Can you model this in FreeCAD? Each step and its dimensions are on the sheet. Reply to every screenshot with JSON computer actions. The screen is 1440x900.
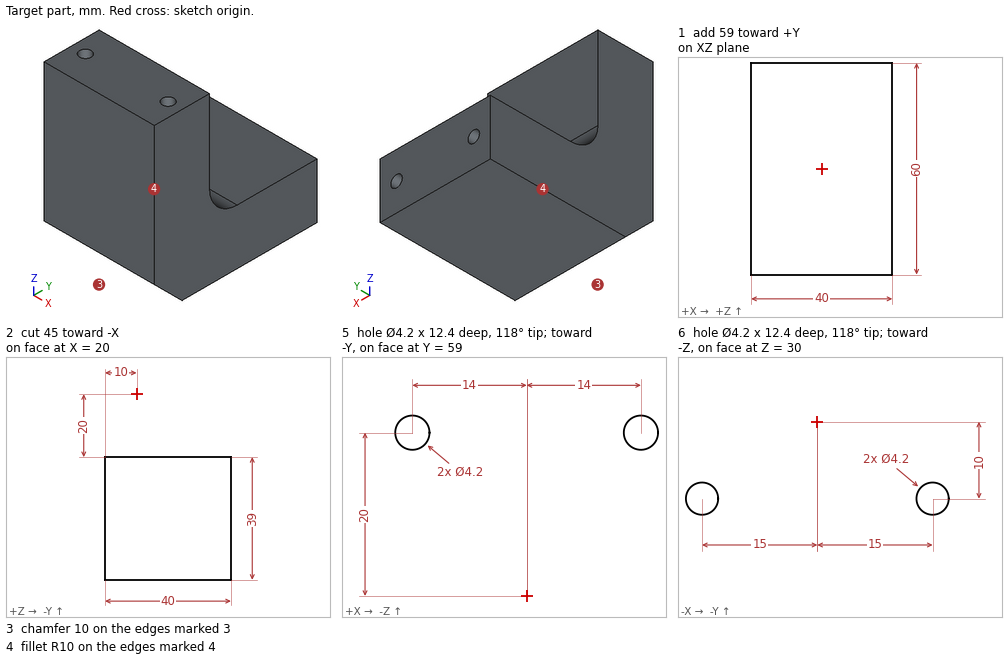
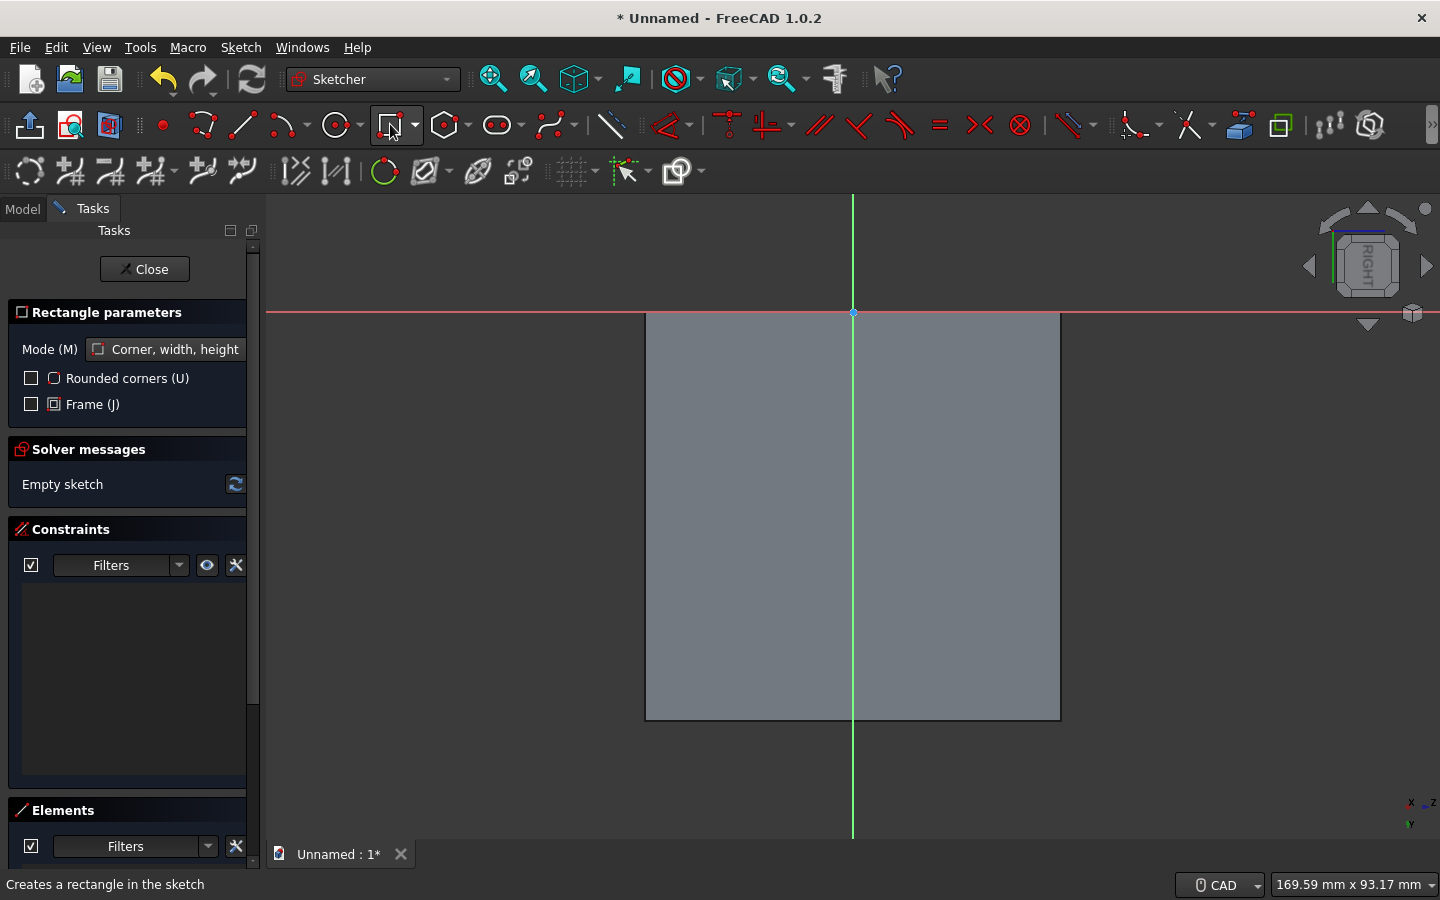
{"action": "left_click", "coordinate": [784, 451]}
{"action": "mouse_move", "coordinate": [1061, 721]}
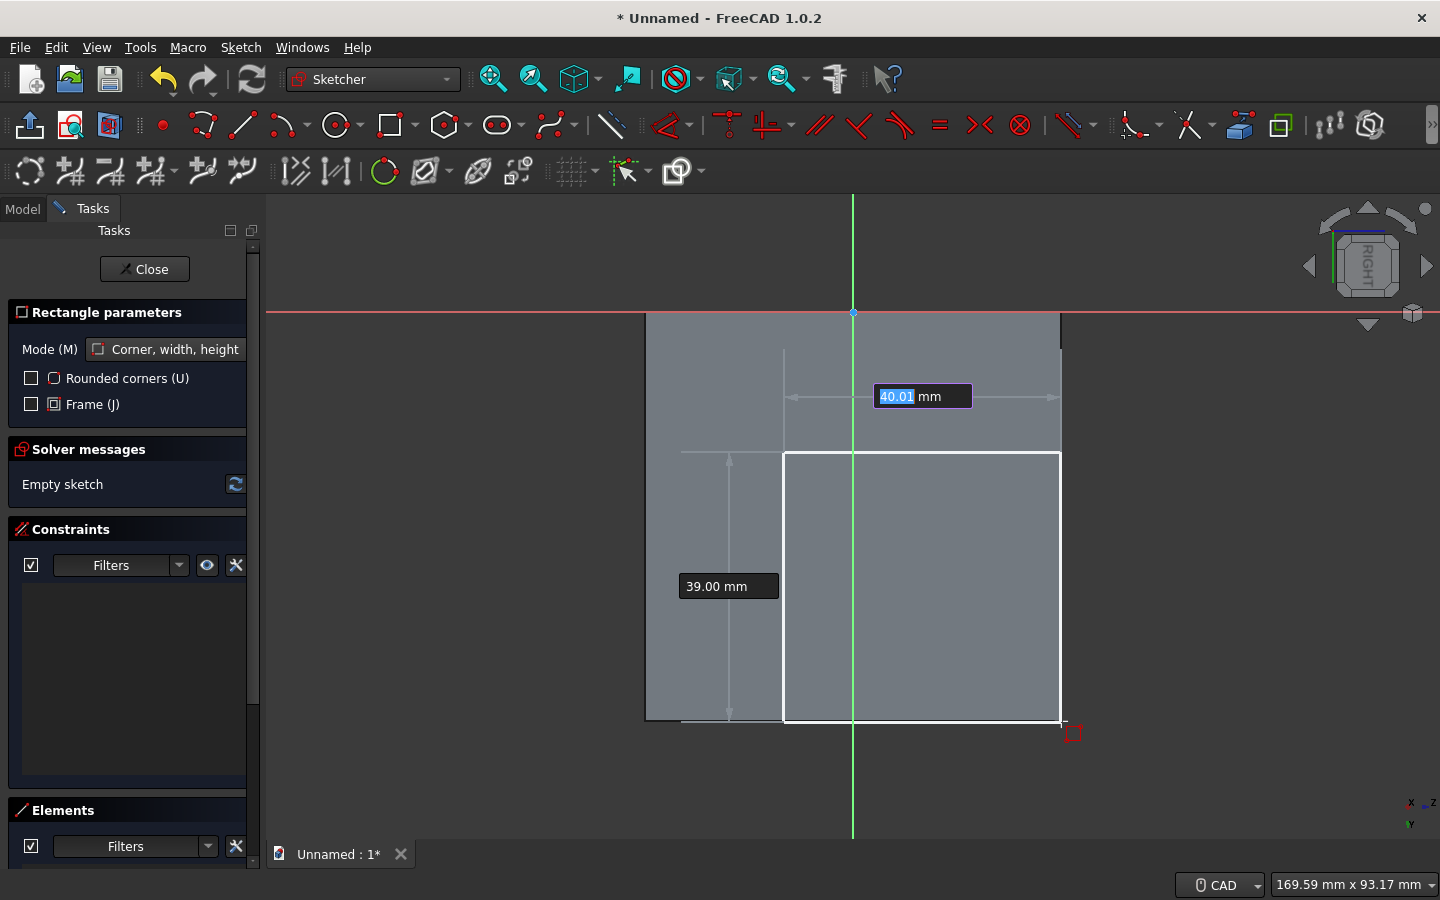
{"action": "type", "text": "40"}
{"action": "key", "text": "Tab"}
{"action": "type", "text": "39"}
{"action": "key", "text": "Return"}
{"action": "key", "text": "Escape"}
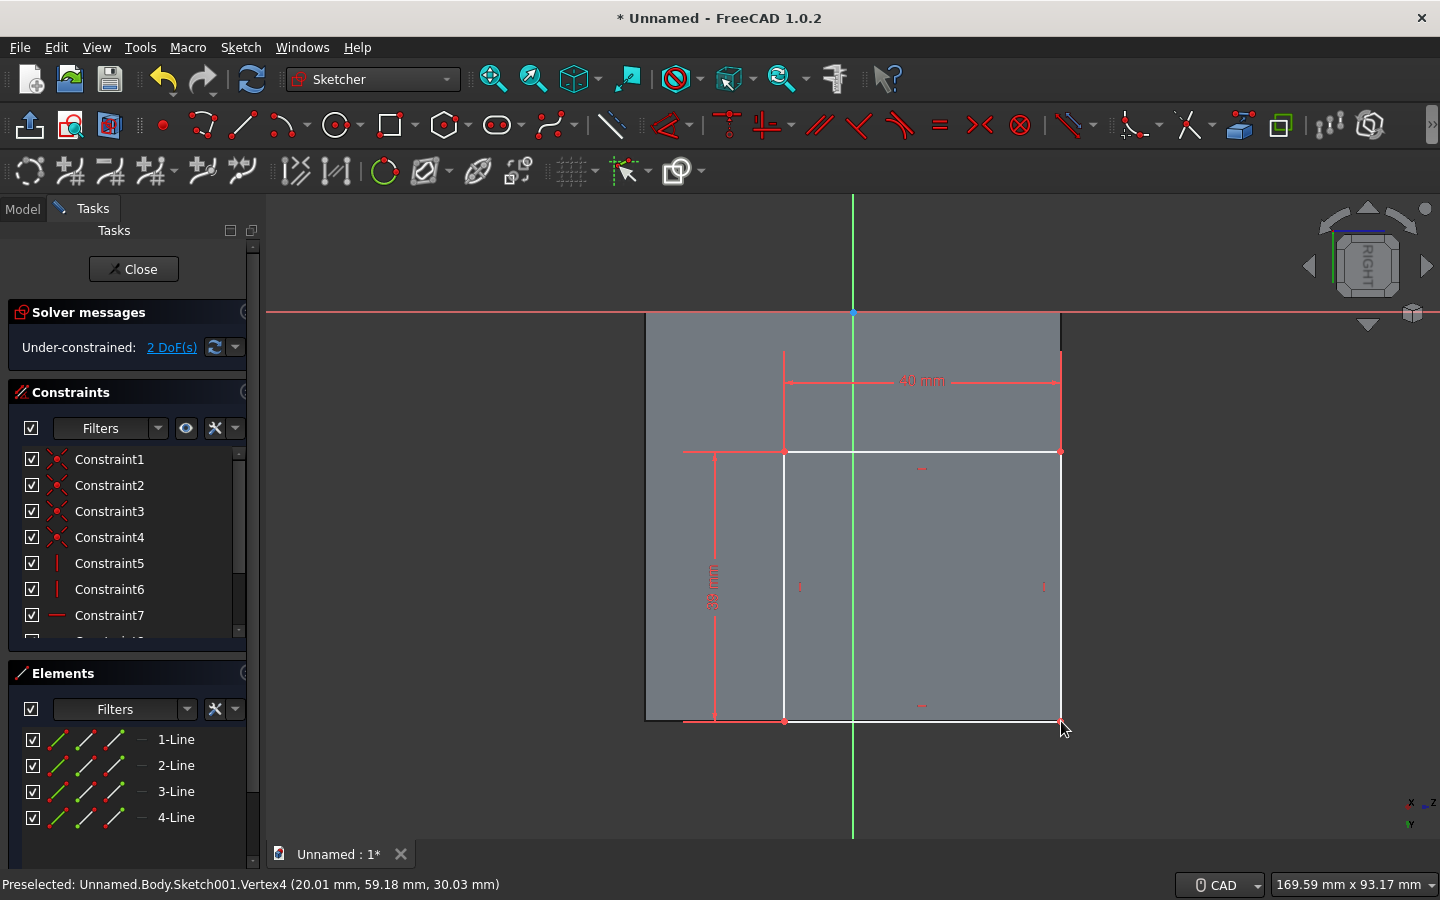
{"action": "left_click", "coordinate": [666, 126]}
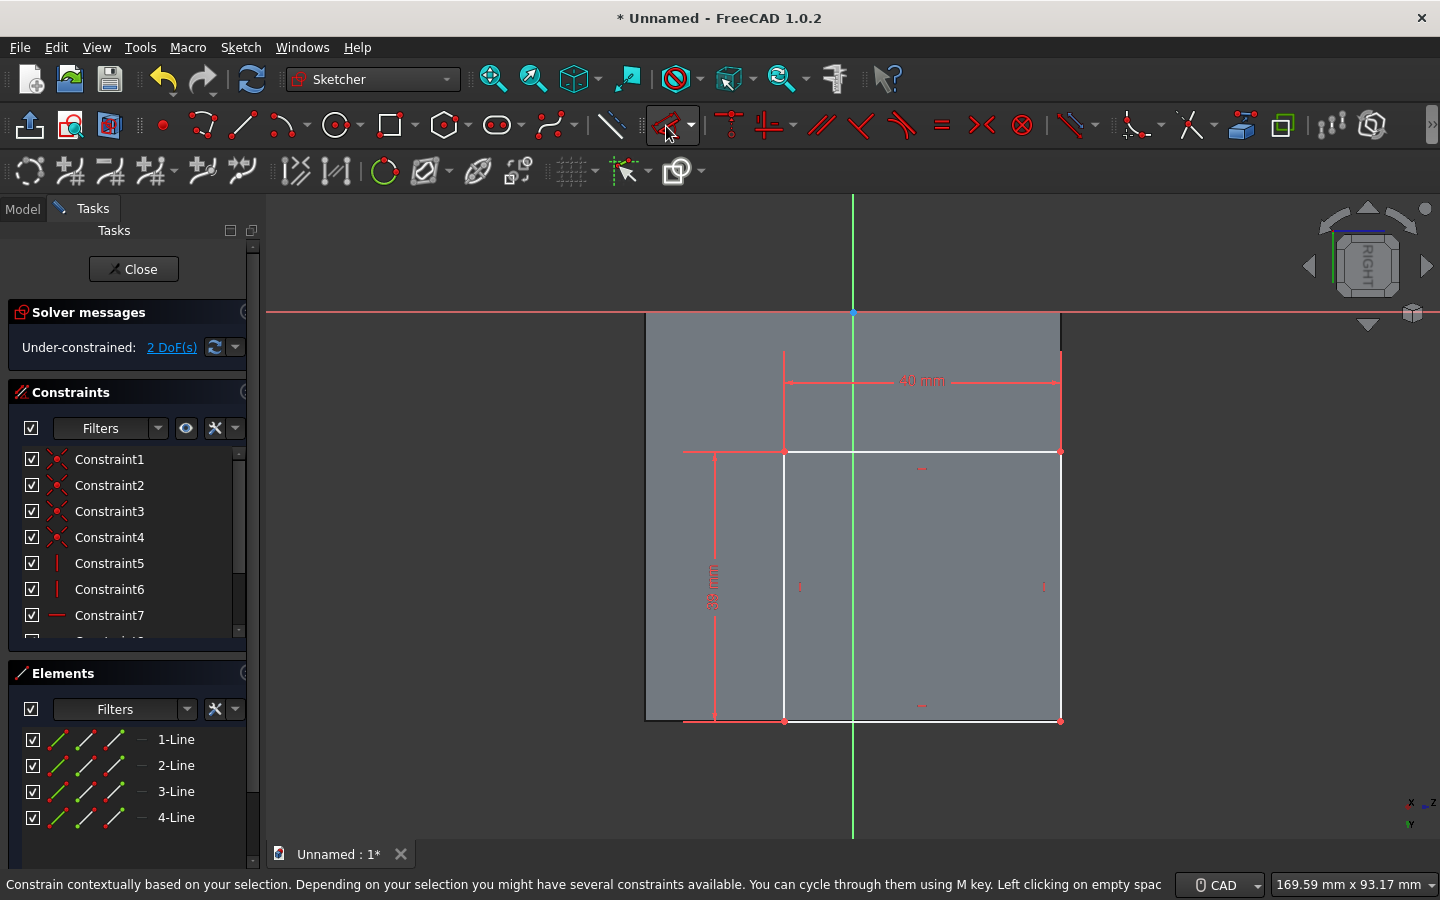
{"action": "left_click", "coordinate": [784, 452]}
{"action": "left_click", "coordinate": [818, 278]}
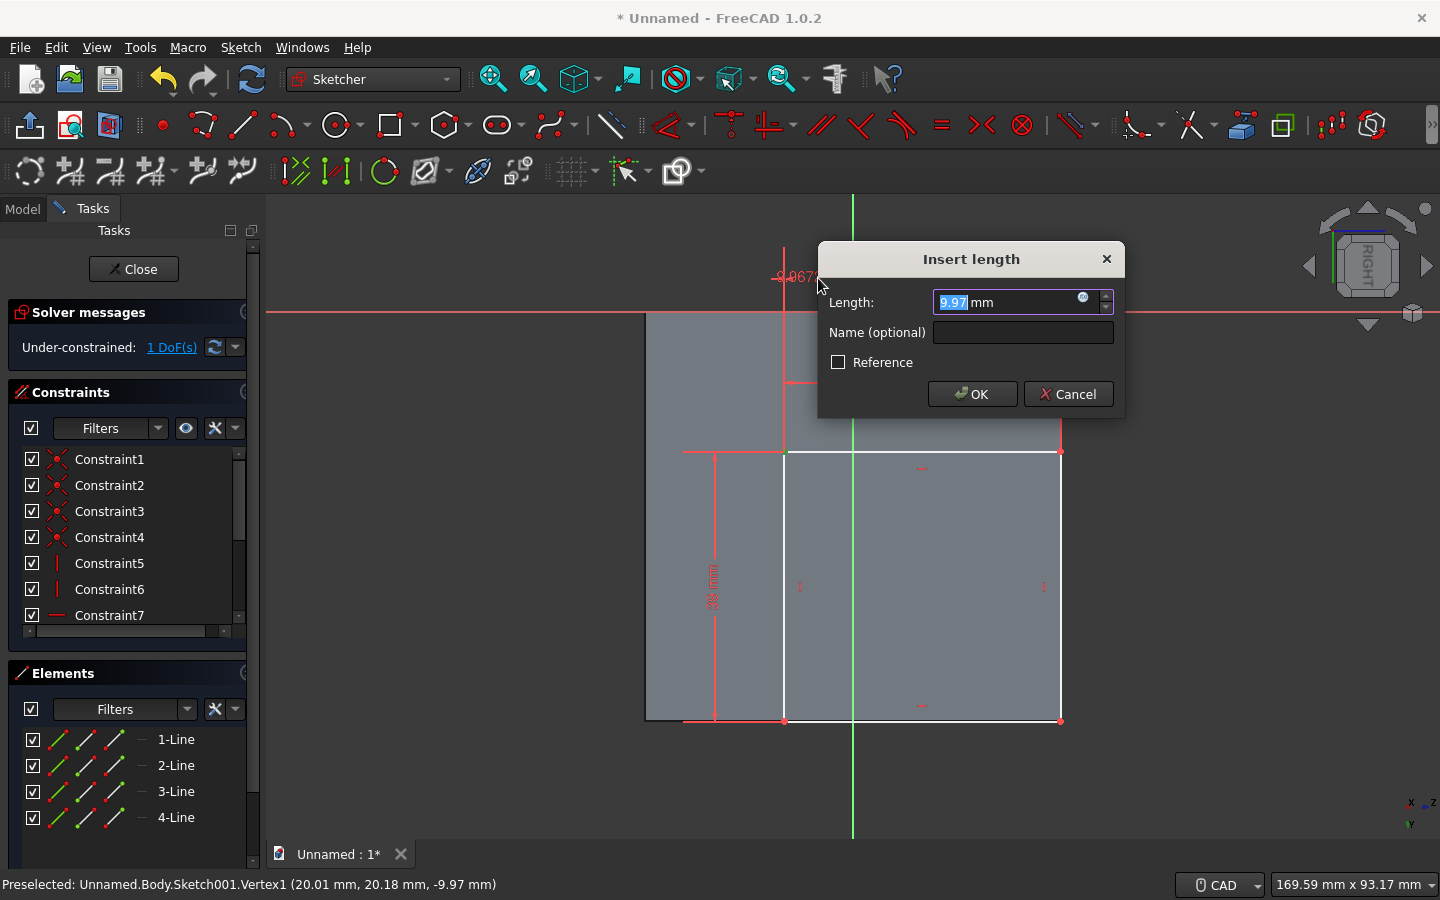
{"action": "type", "text": "10"}
{"action": "key", "text": "Return"}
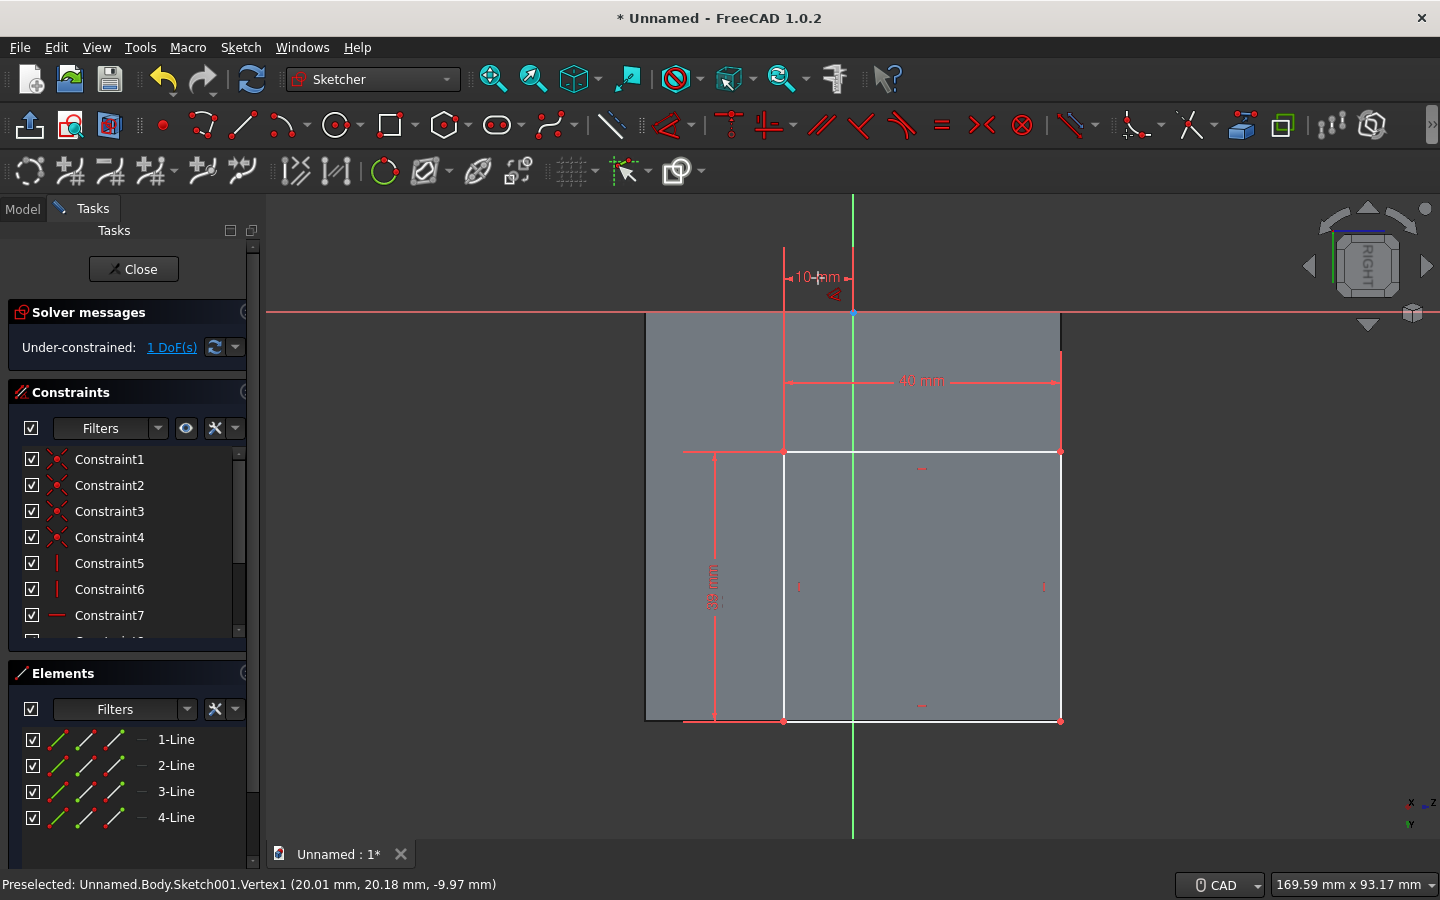
{"action": "left_click", "coordinate": [784, 452]}
{"action": "left_click", "coordinate": [750, 382]}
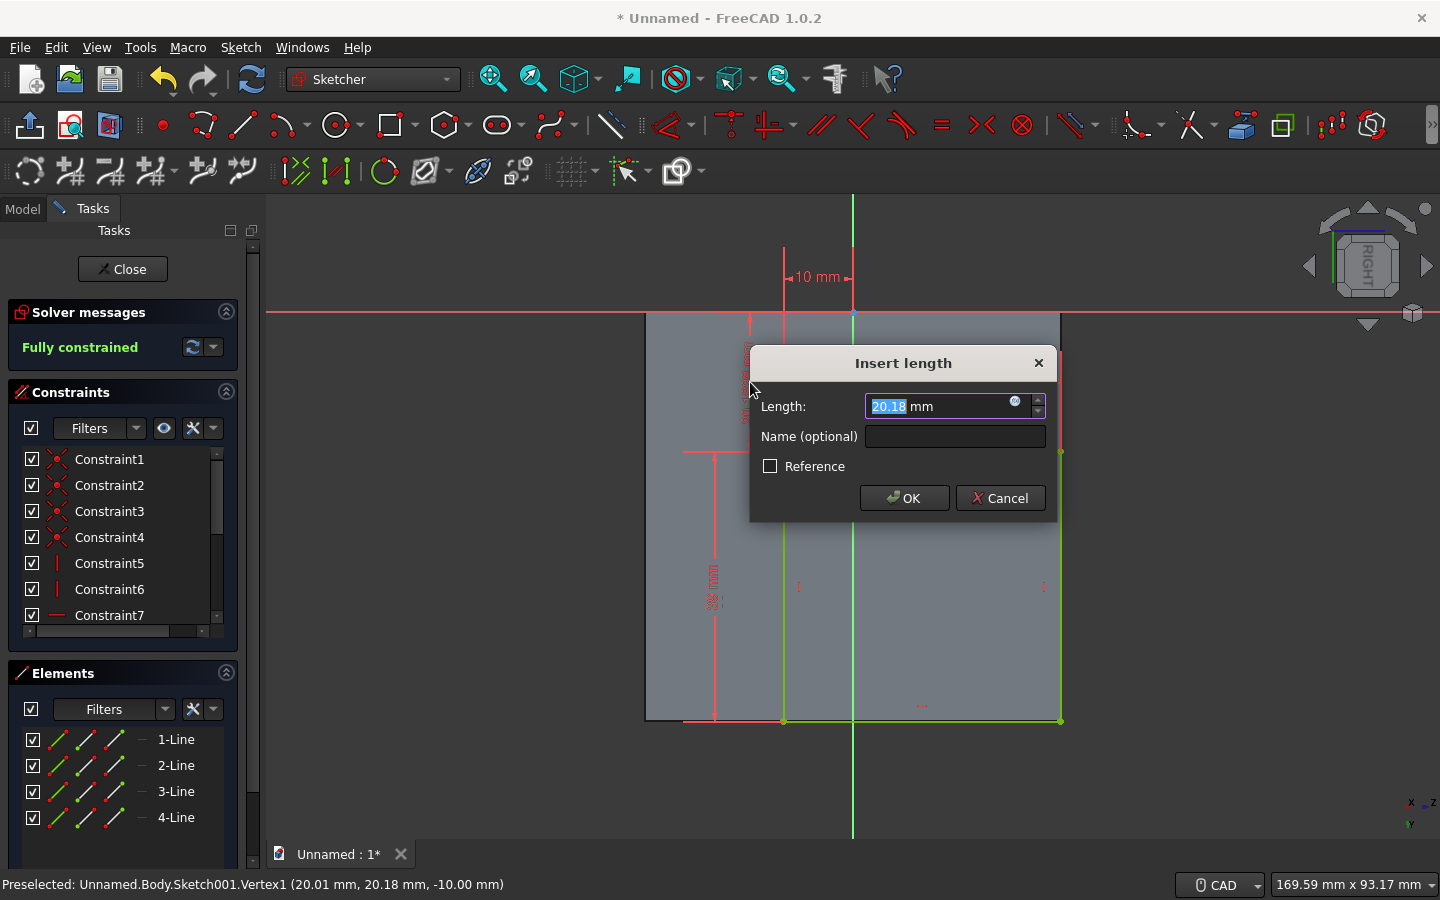
{"action": "type", "text": "20"}
{"action": "key", "text": "Return"}
{"action": "key", "text": "Escape"}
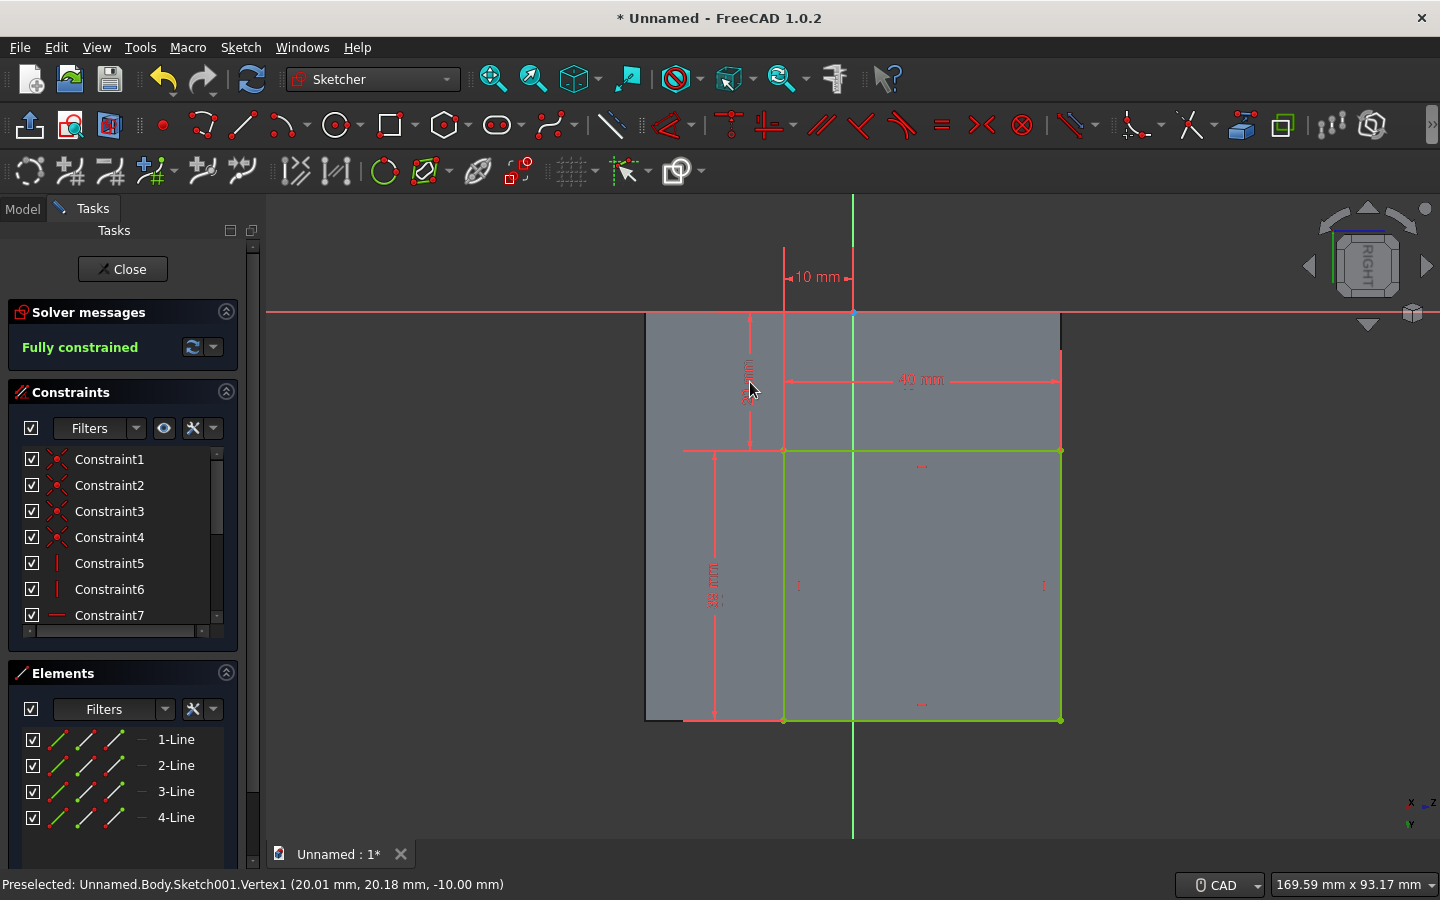
{"action": "left_click", "coordinate": [123, 269]}